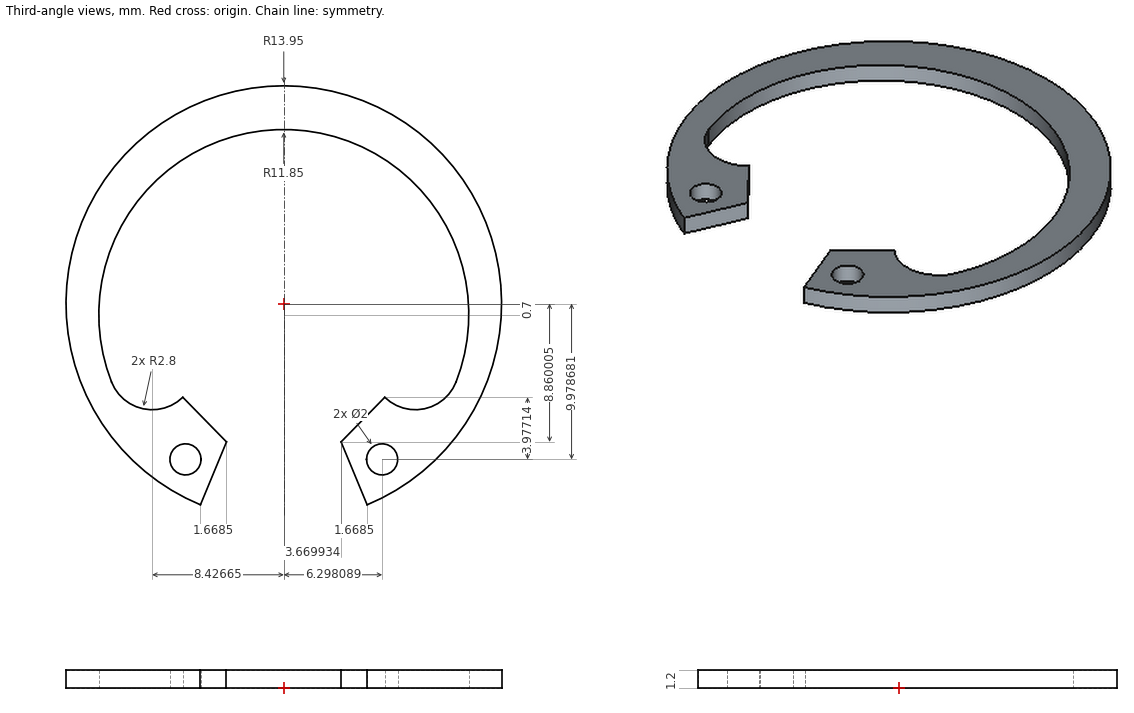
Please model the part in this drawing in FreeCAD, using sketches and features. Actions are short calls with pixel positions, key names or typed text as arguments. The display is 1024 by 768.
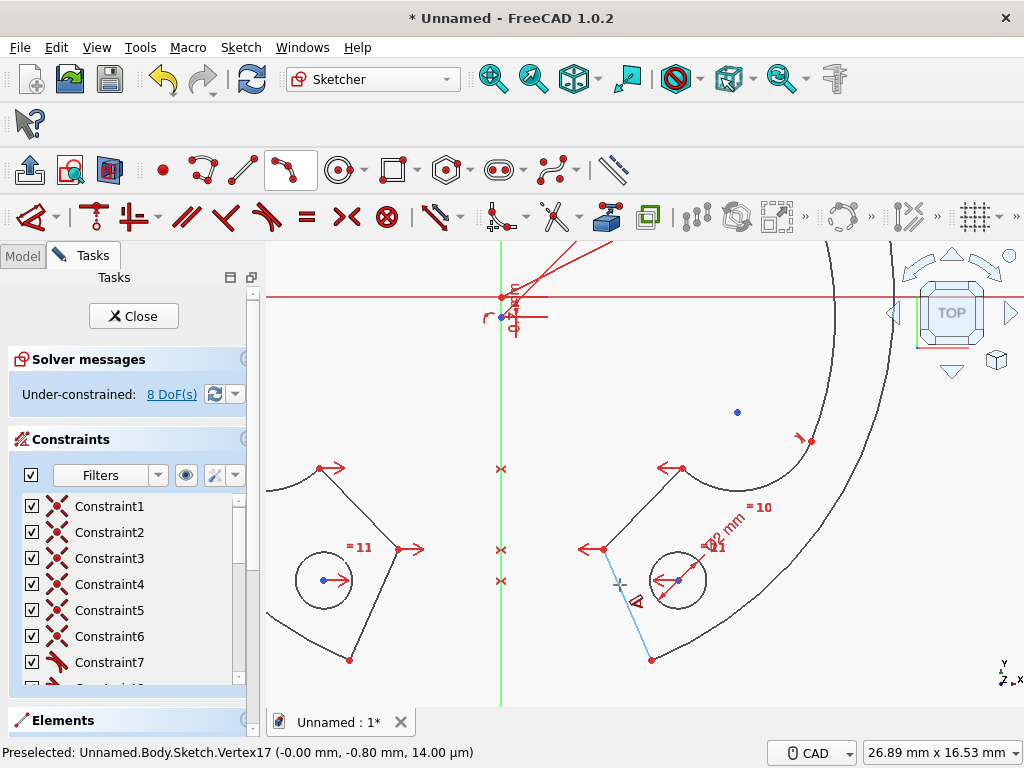
click(618, 583)
click(616, 515)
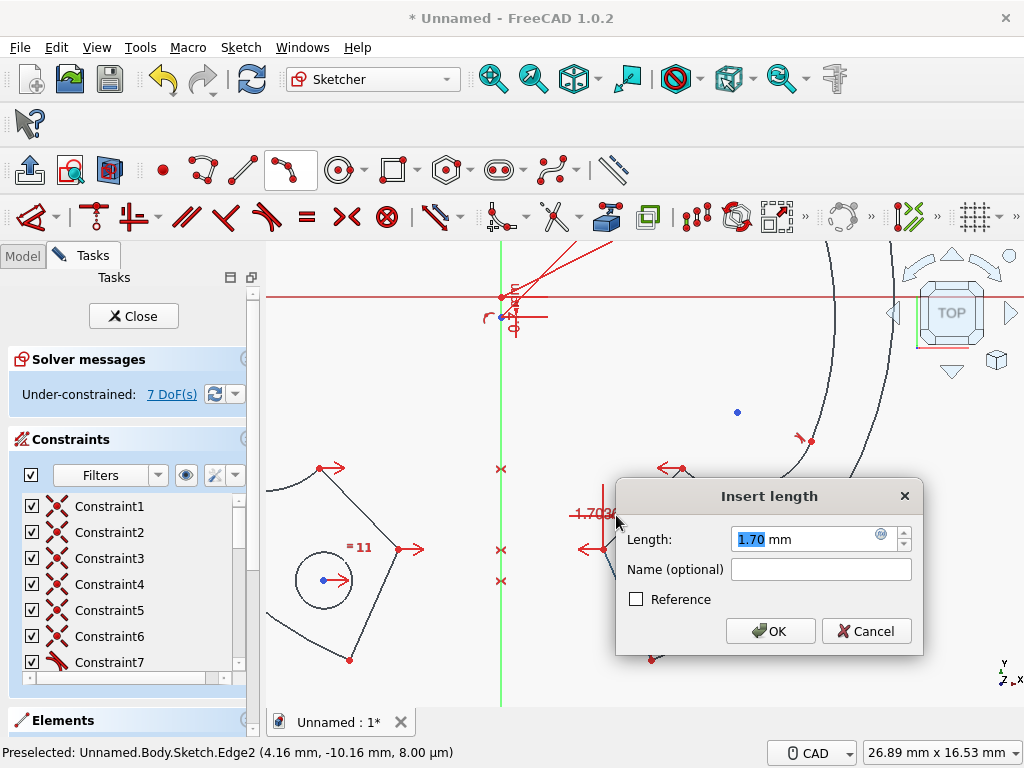
text(1.6685)
key(Return)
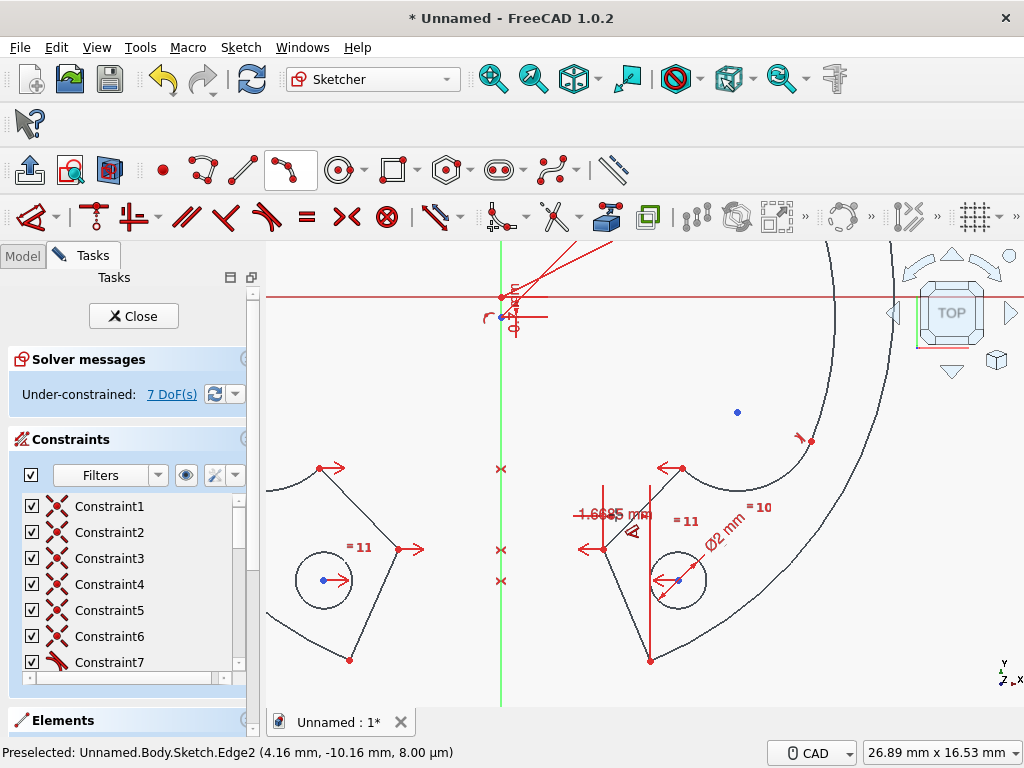
click(364, 627)
click(385, 515)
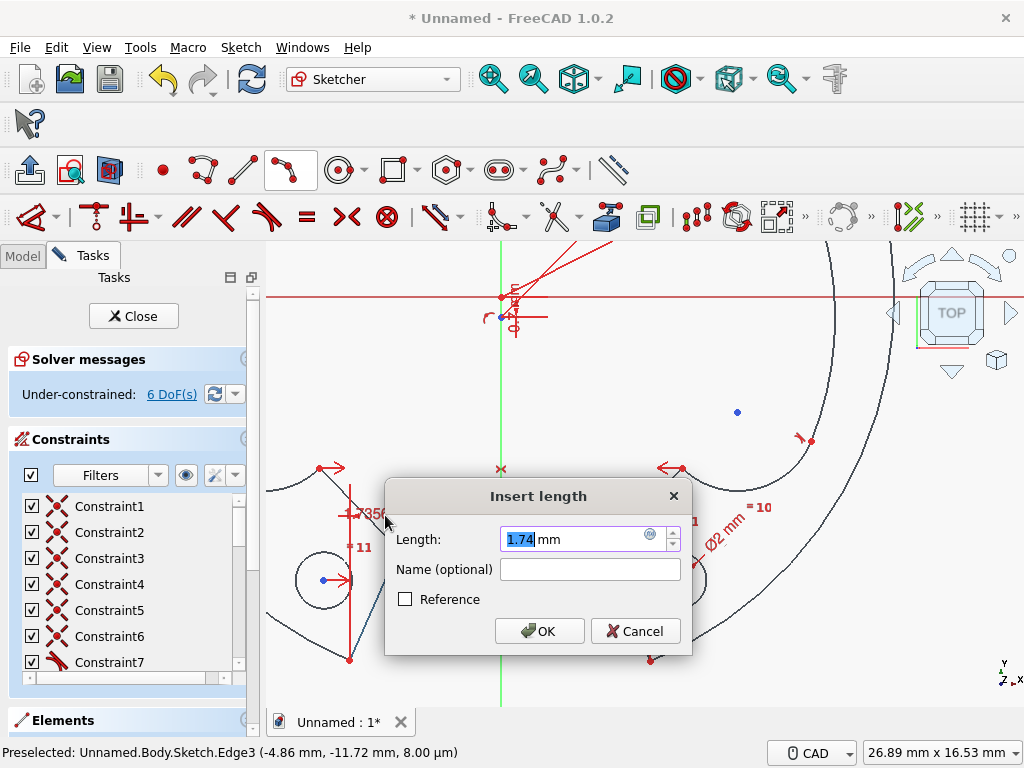
text(1.6685)
key(Return)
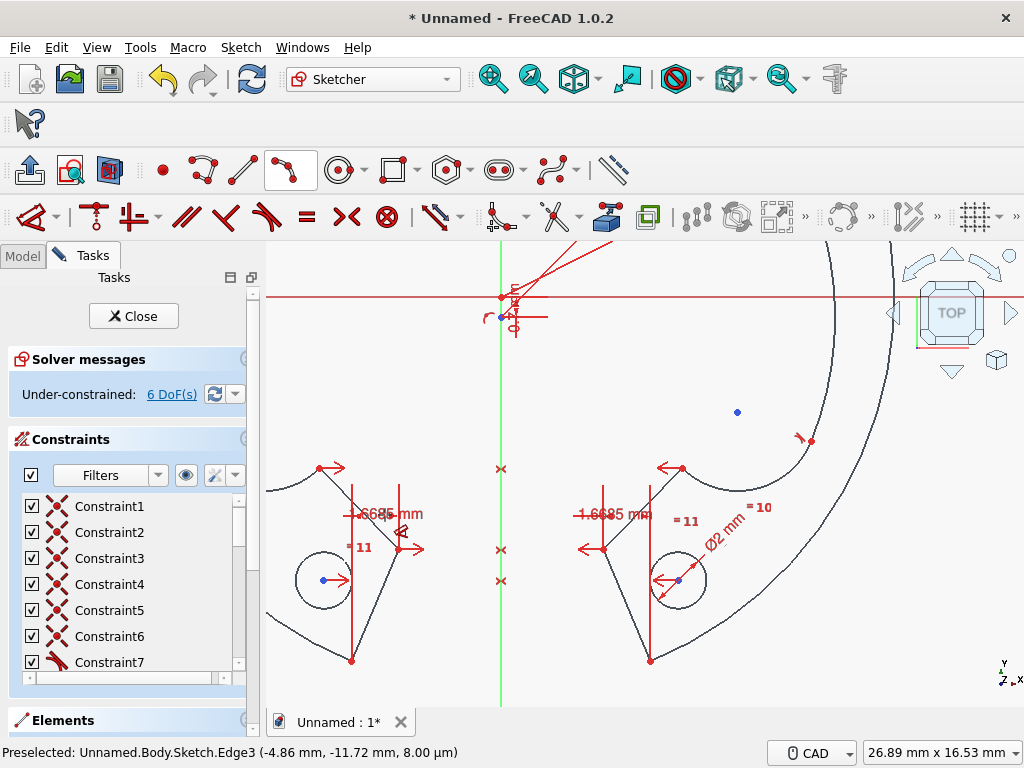
scroll(620, 585, down, 5)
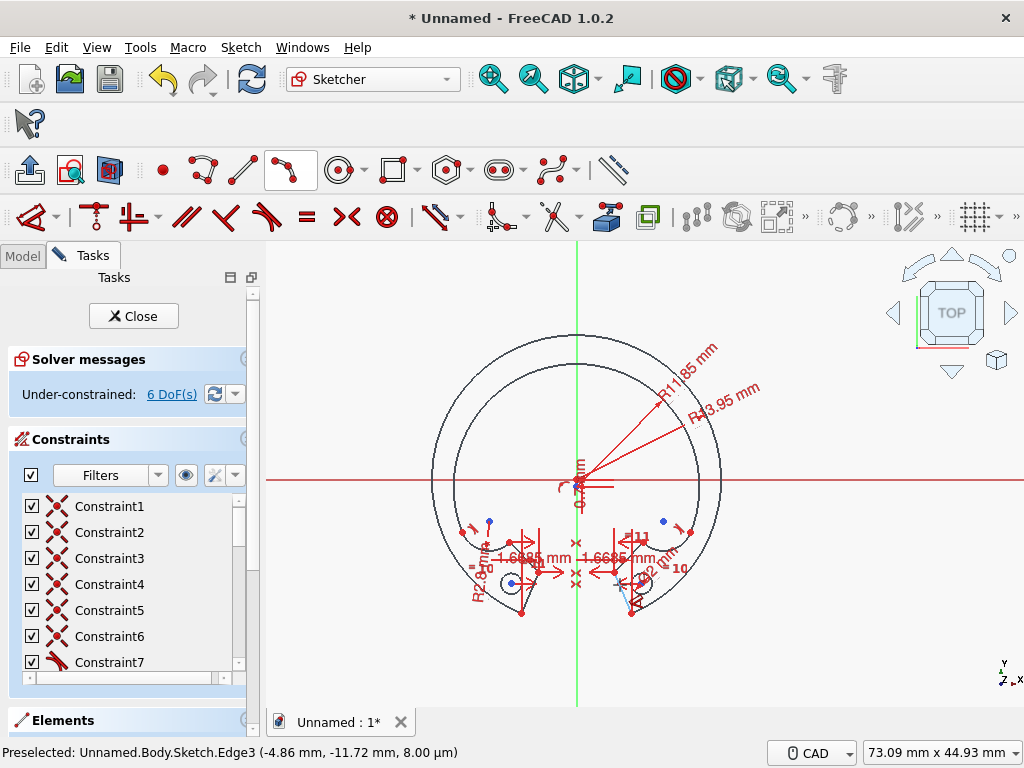
click(489, 522)
click(533, 446)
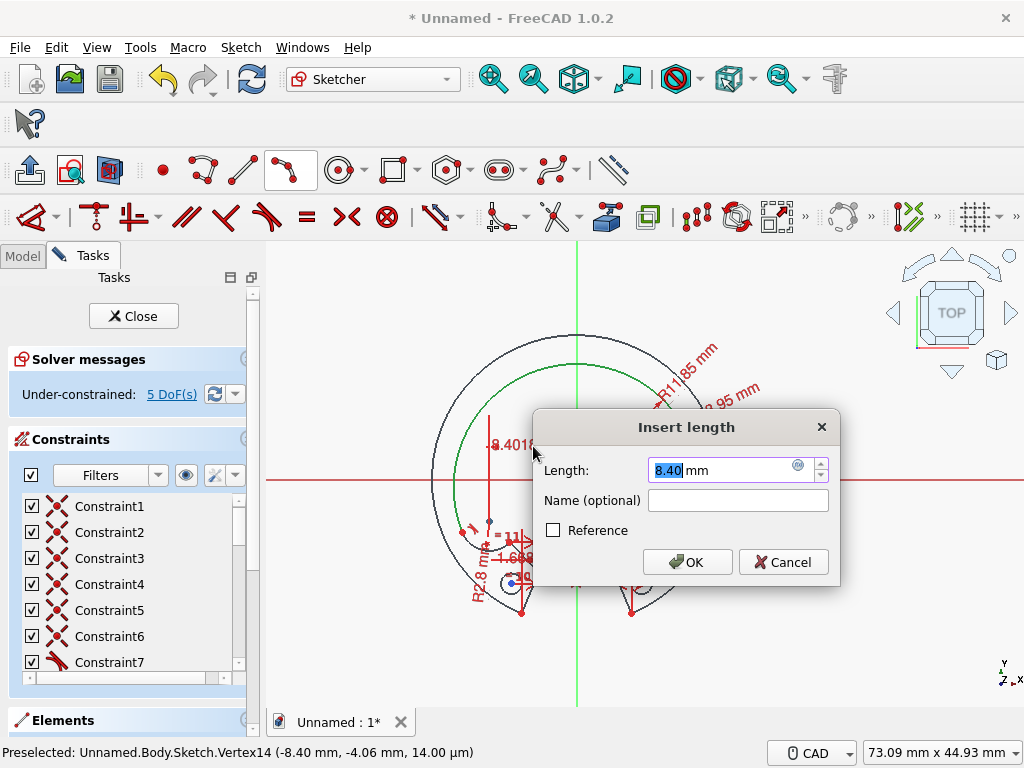
text(8.42665)
key(Return)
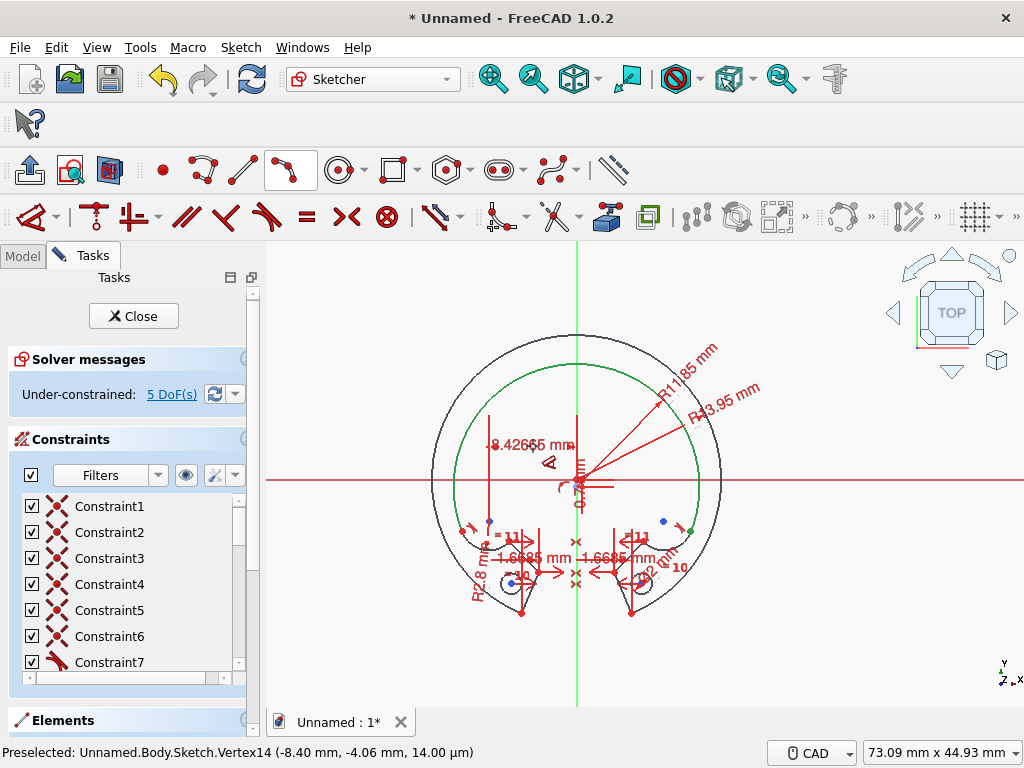
click(642, 584)
click(609, 618)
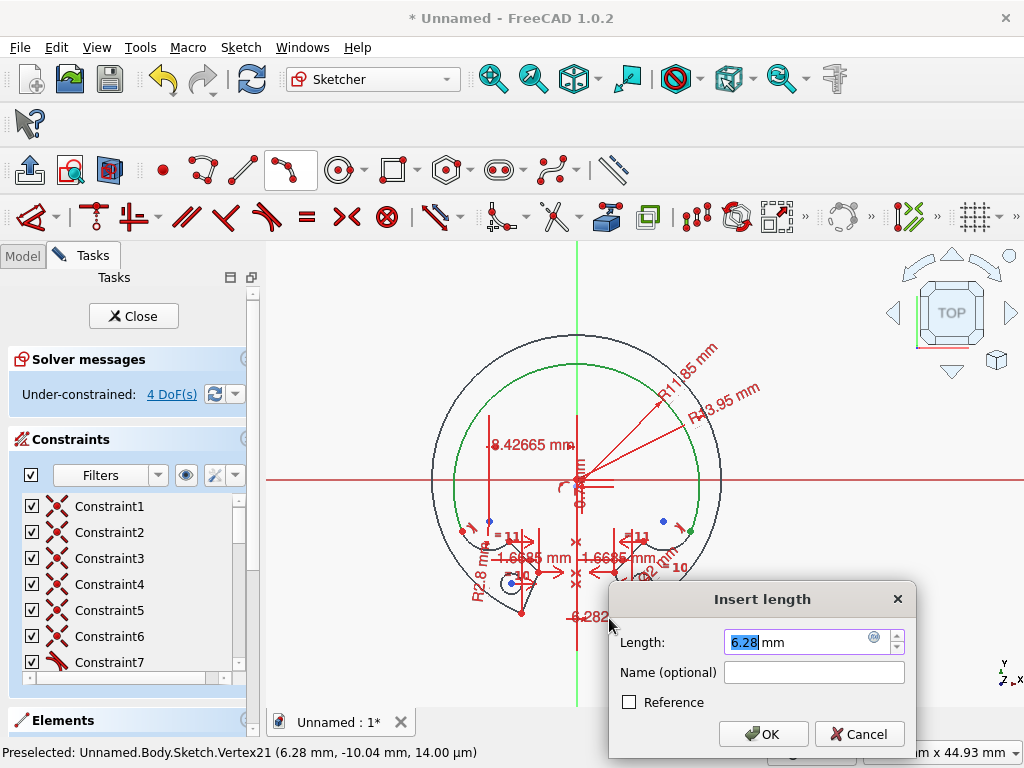
text(6.298089)
key(Return)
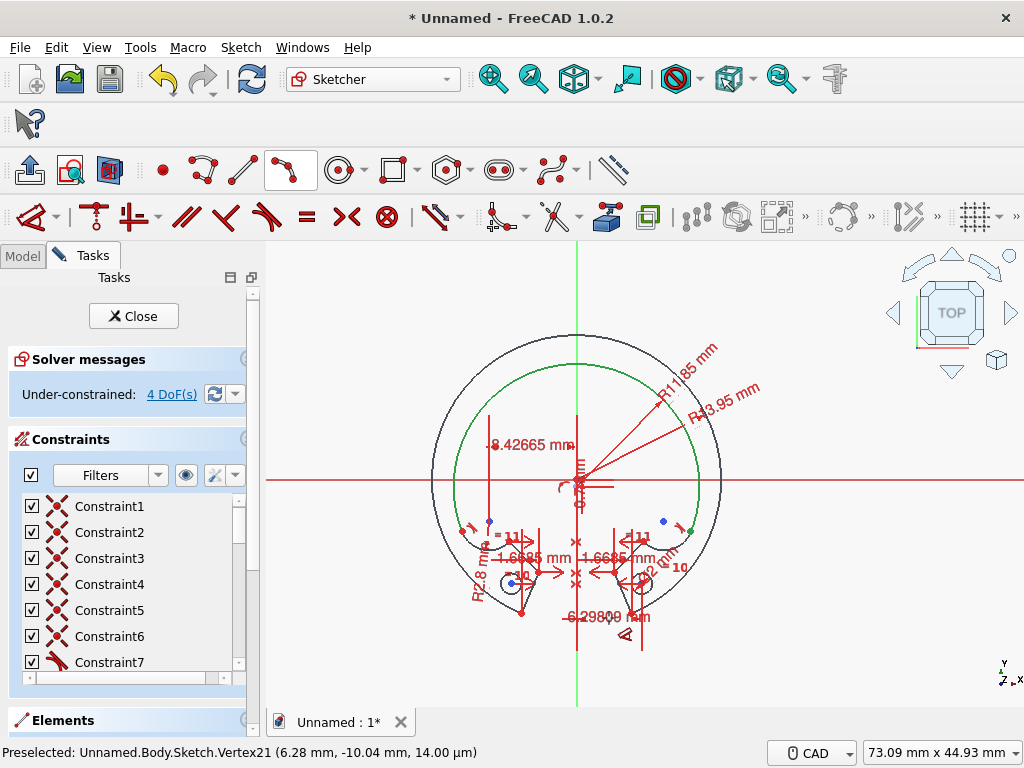
click(642, 584)
click(676, 532)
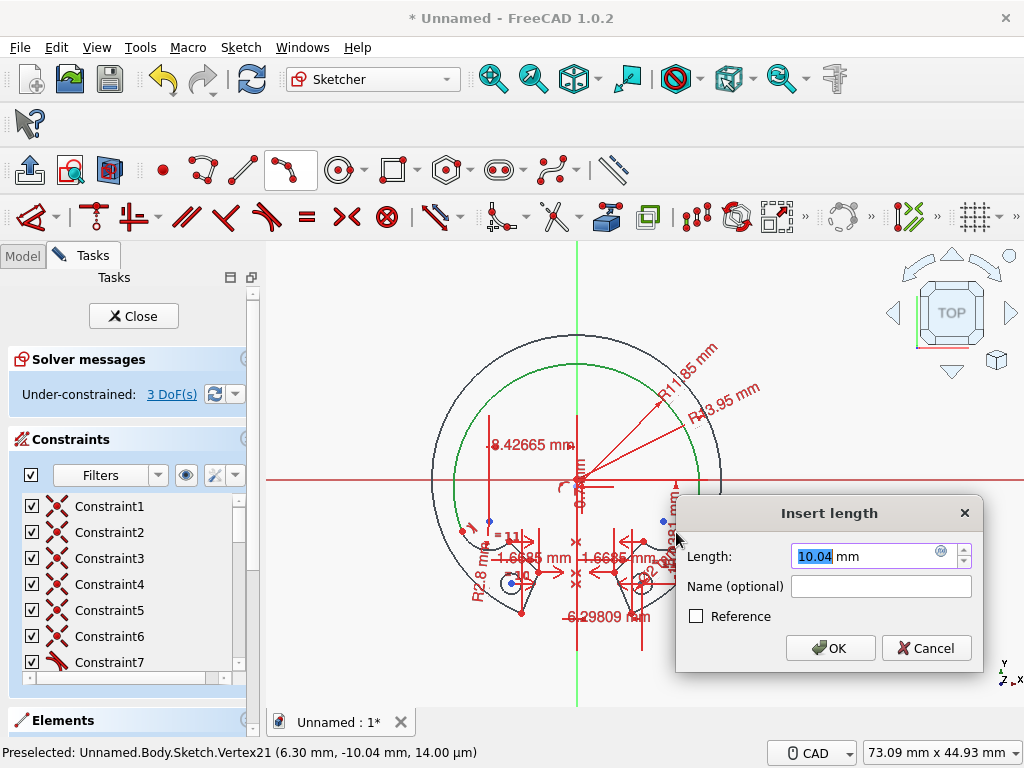
text(9.978681)
key(Return)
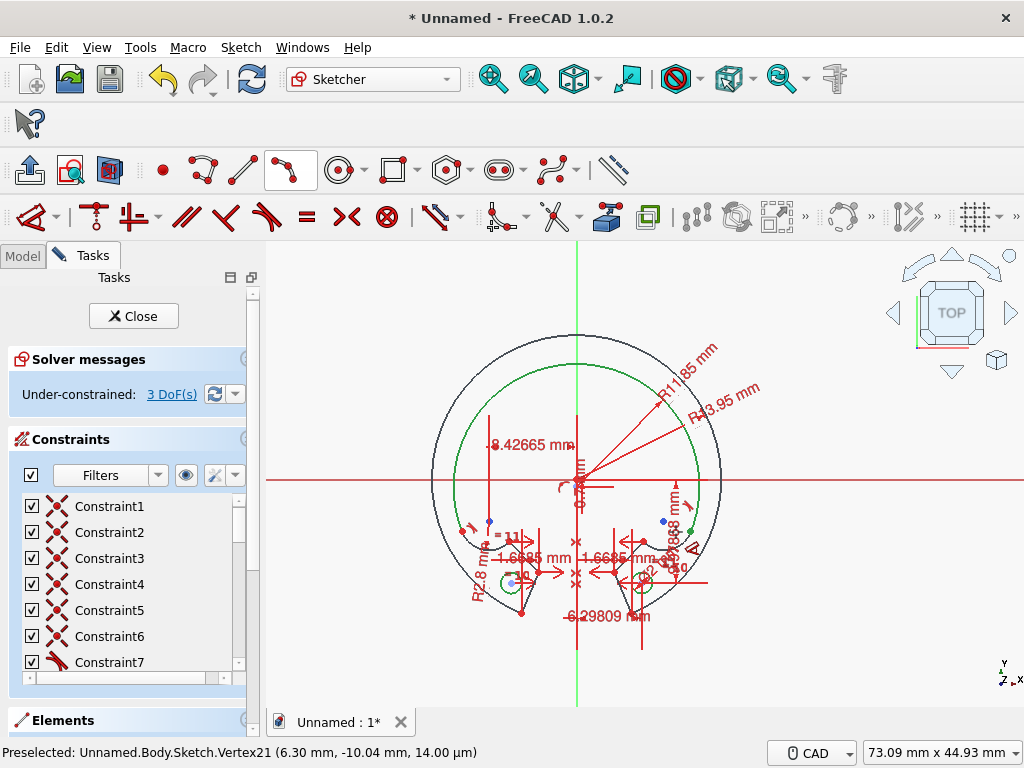
click(644, 542)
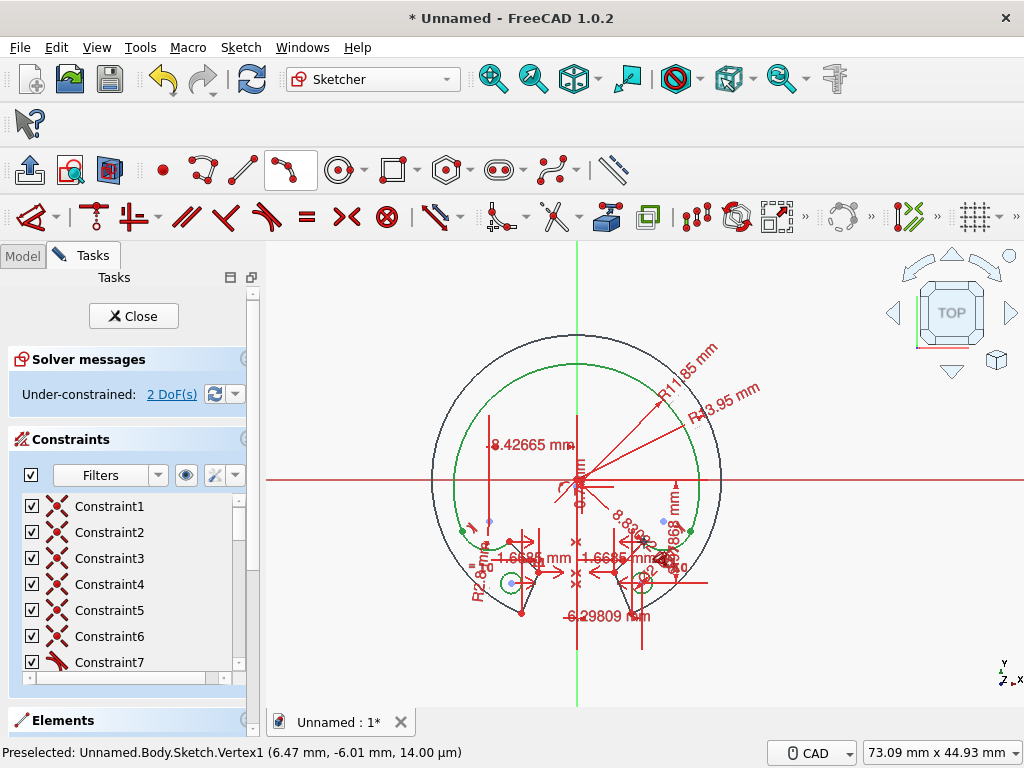
click(642, 583)
click(750, 563)